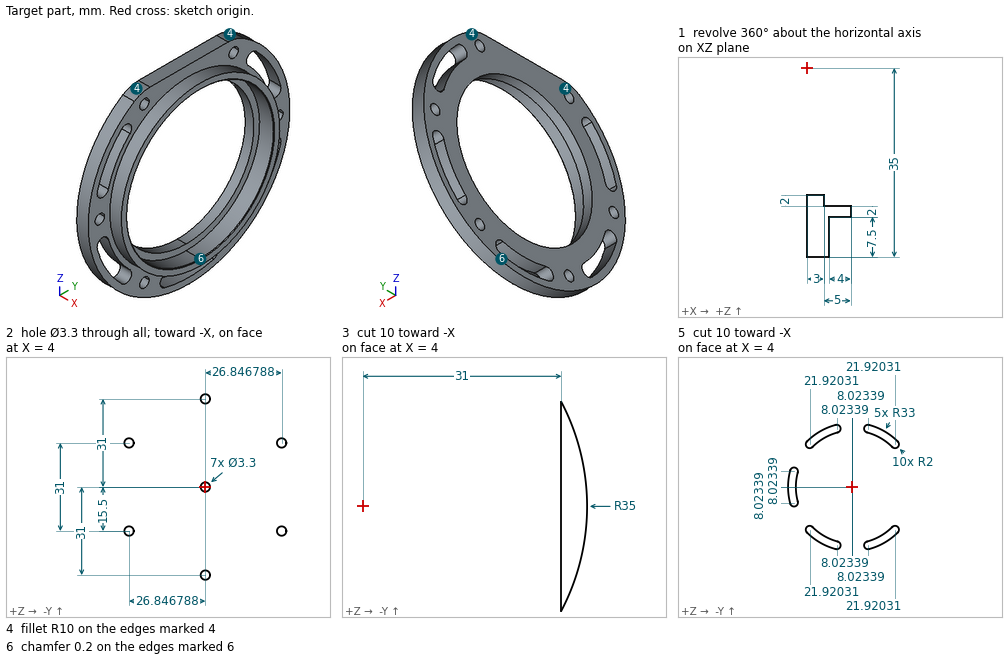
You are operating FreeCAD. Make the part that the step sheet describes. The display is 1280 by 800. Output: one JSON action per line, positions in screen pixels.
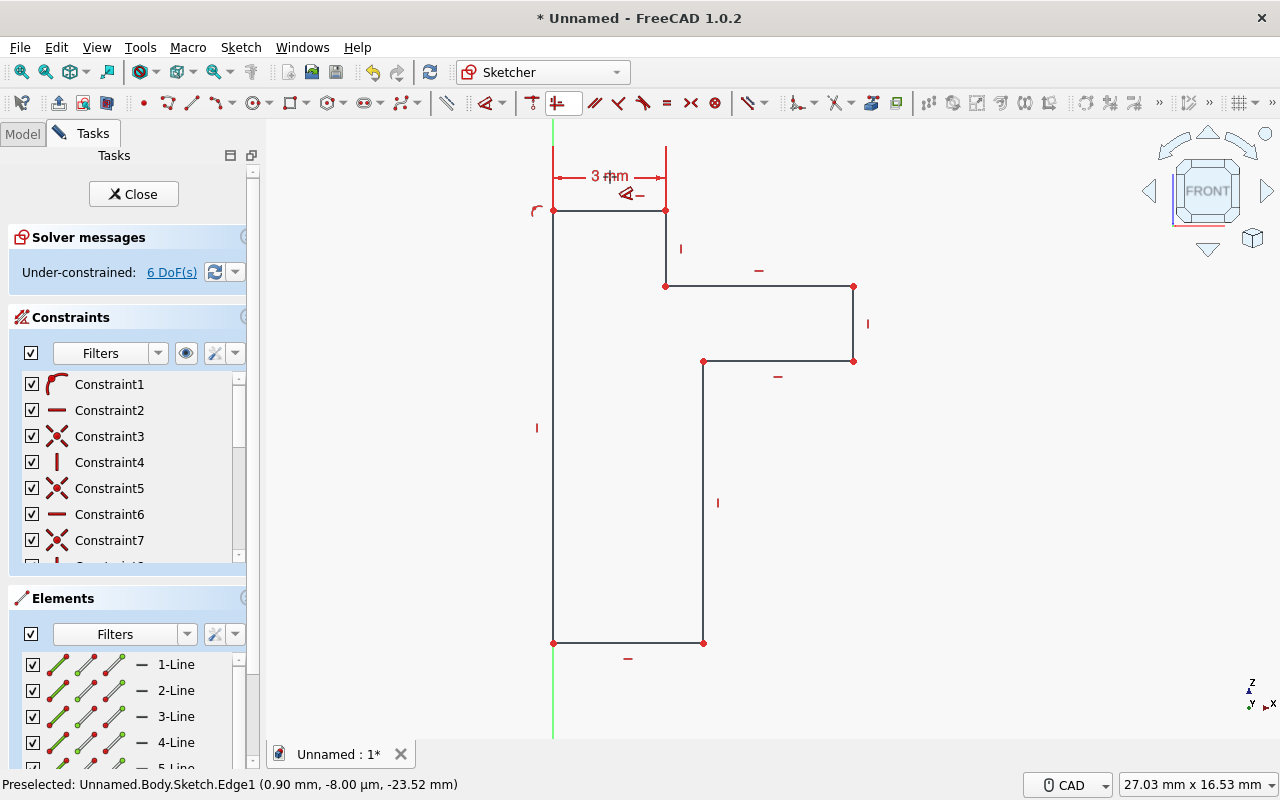
{"action": "left_click", "coordinate": [666, 233]}
{"action": "left_click", "coordinate": [632, 248]}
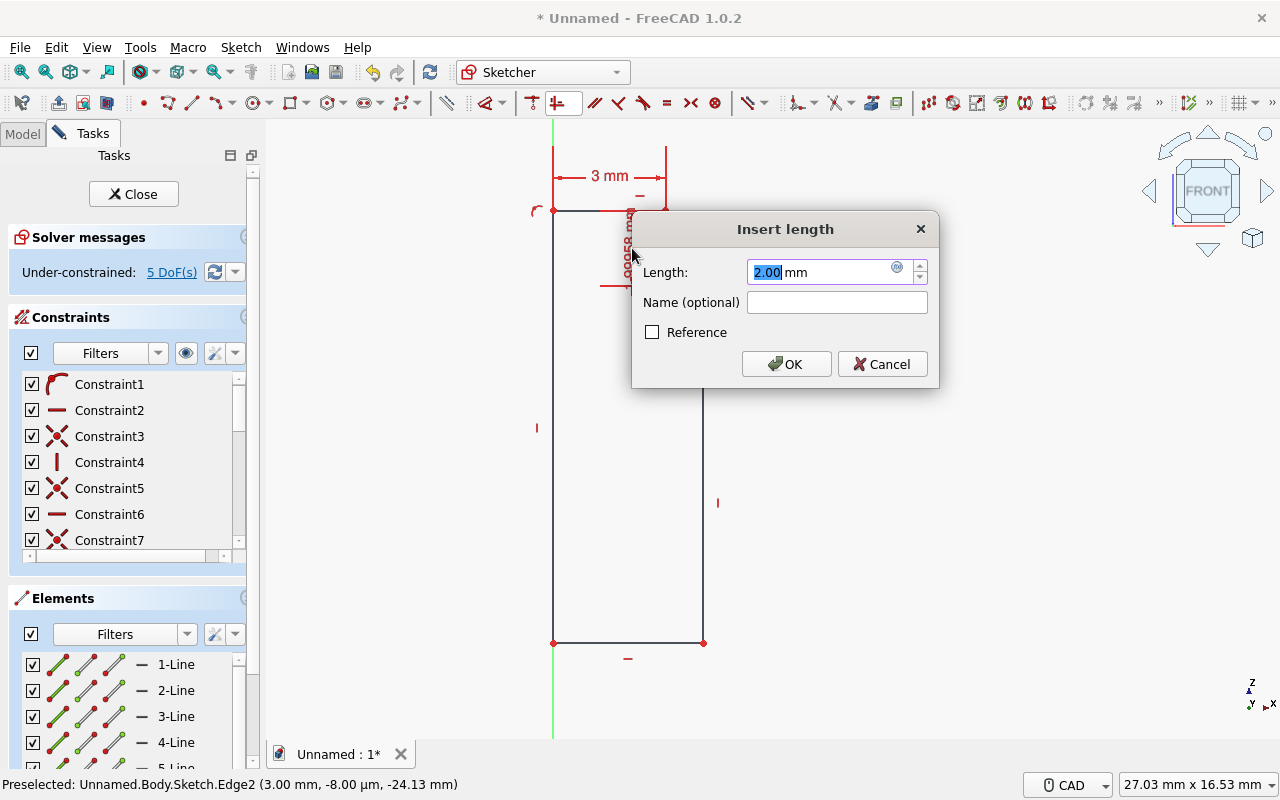
{"action": "type", "text": "2"}
{"action": "key", "text": "Return"}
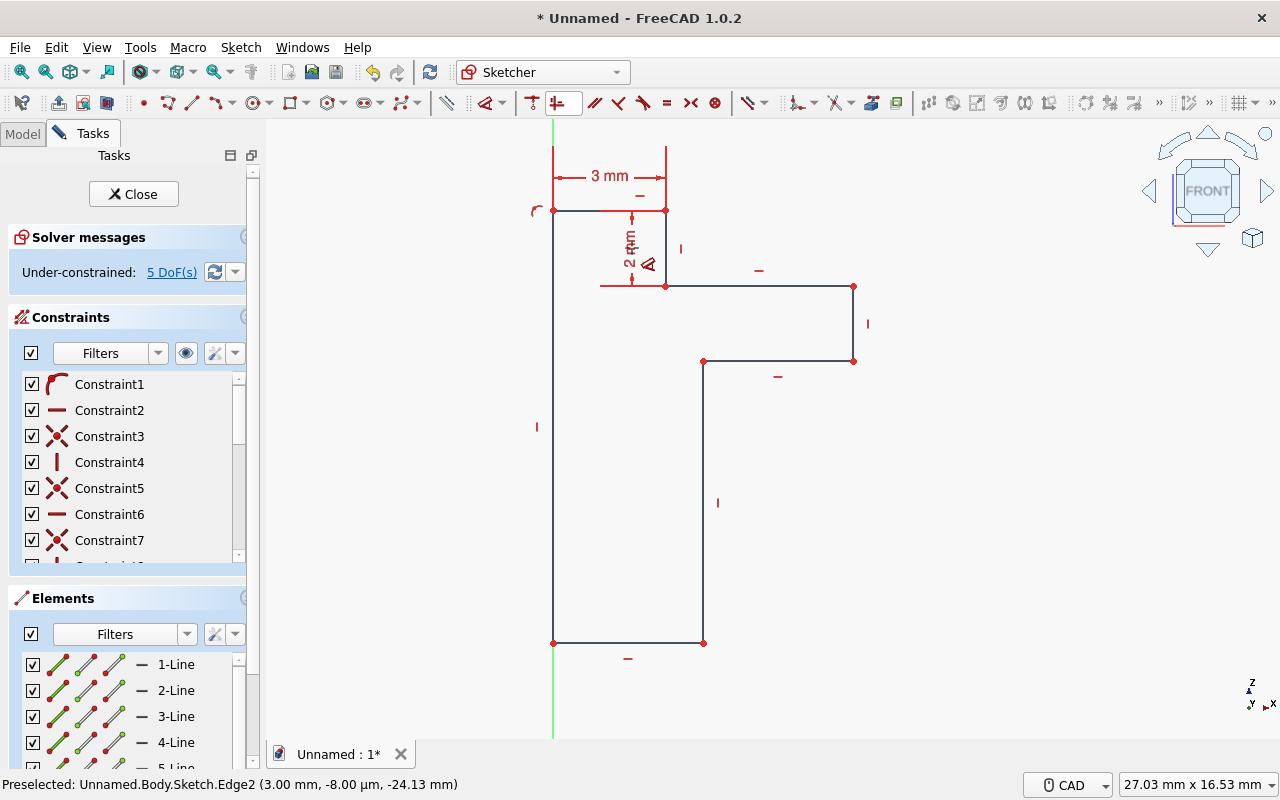
{"action": "left_click", "coordinate": [722, 286]}
{"action": "left_click", "coordinate": [759, 252]}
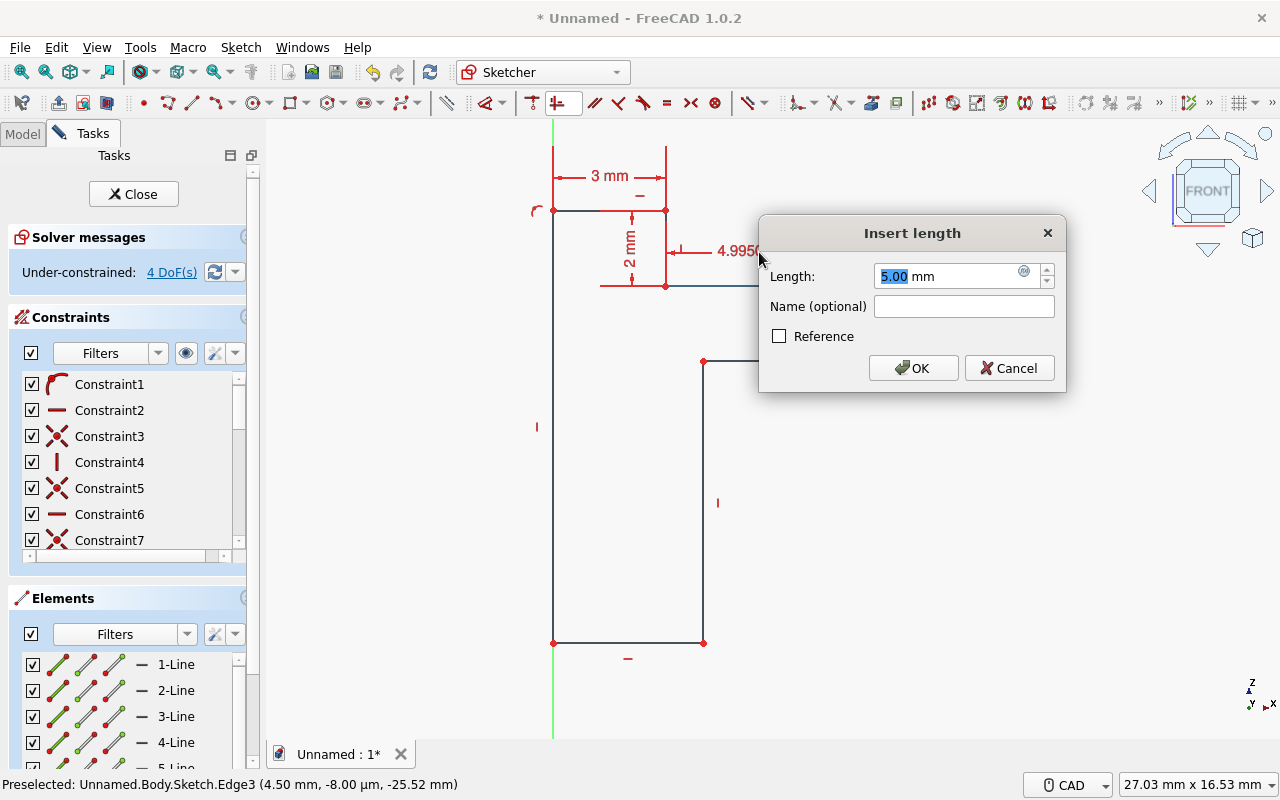
{"action": "type", "text": "5"}
{"action": "key", "text": "Return"}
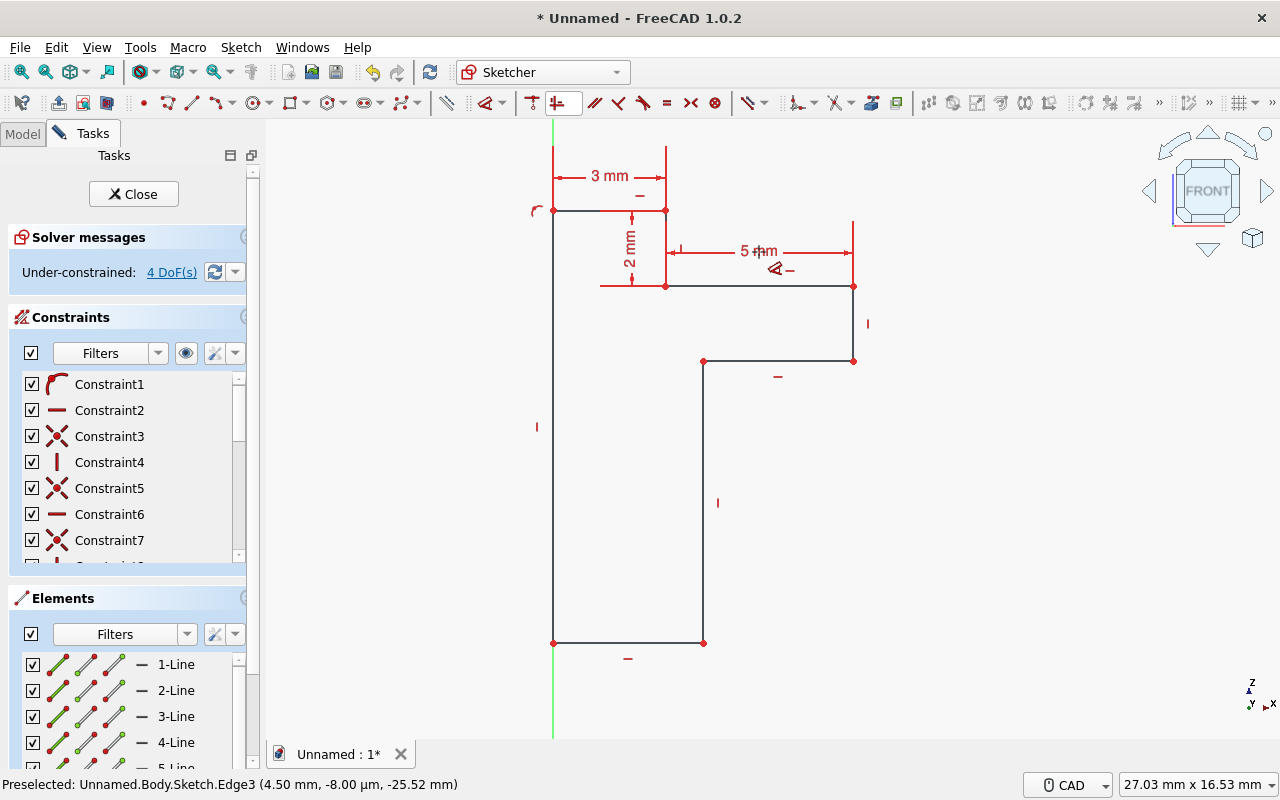
{"action": "left_click", "coordinate": [853, 308]}
{"action": "left_click", "coordinate": [887, 323]}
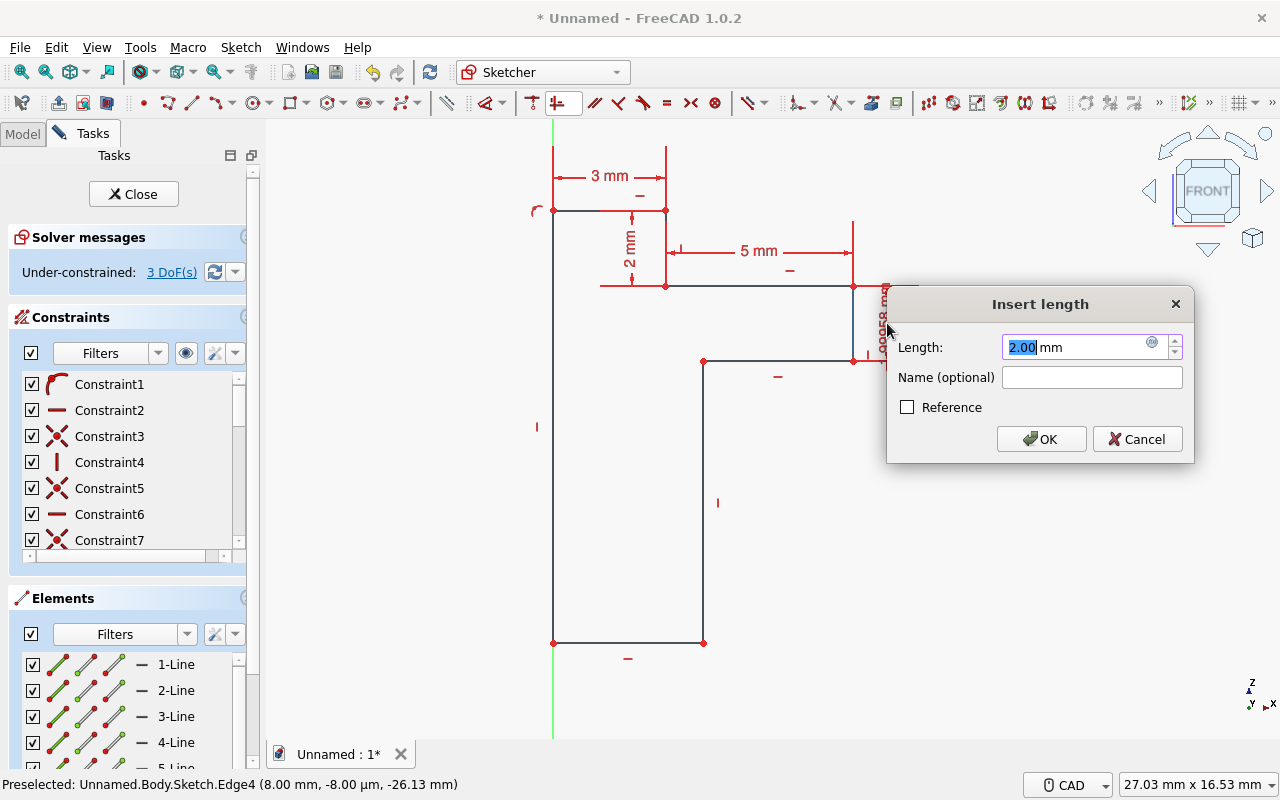
{"action": "type", "text": "2"}
{"action": "key", "text": "Return"}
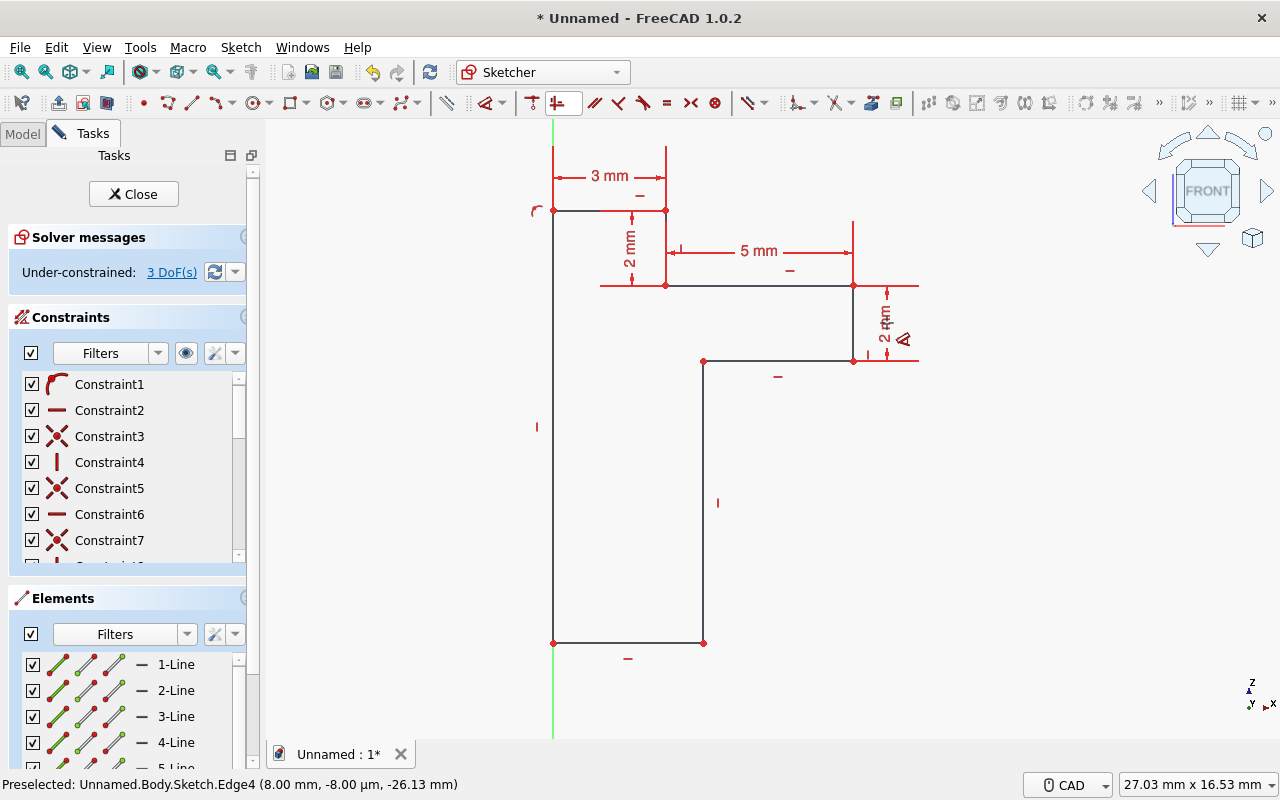
{"action": "left_click", "coordinate": [808, 361]}
{"action": "left_click", "coordinate": [778, 327]}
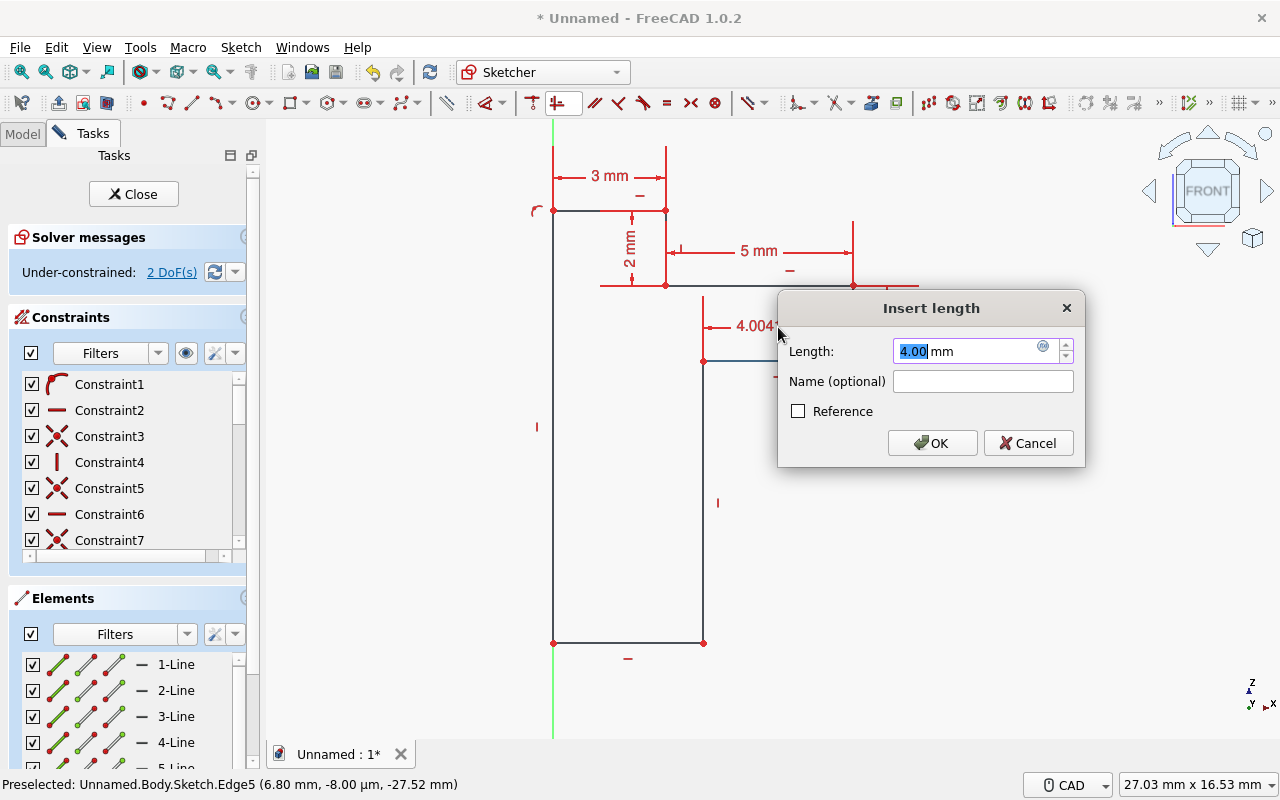
{"action": "type", "text": "4"}
{"action": "key", "text": "Return"}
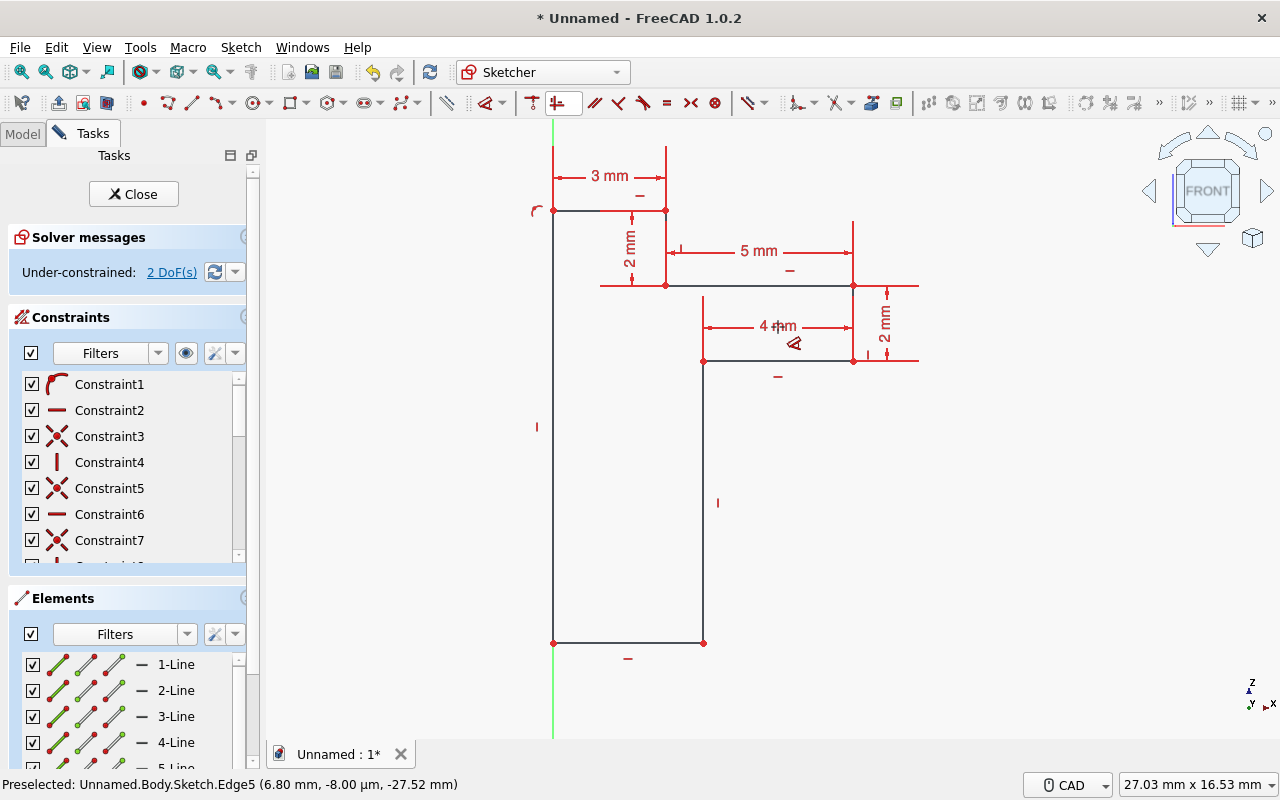
{"action": "left_click", "coordinate": [703, 446]}
{"action": "left_click", "coordinate": [737, 502]}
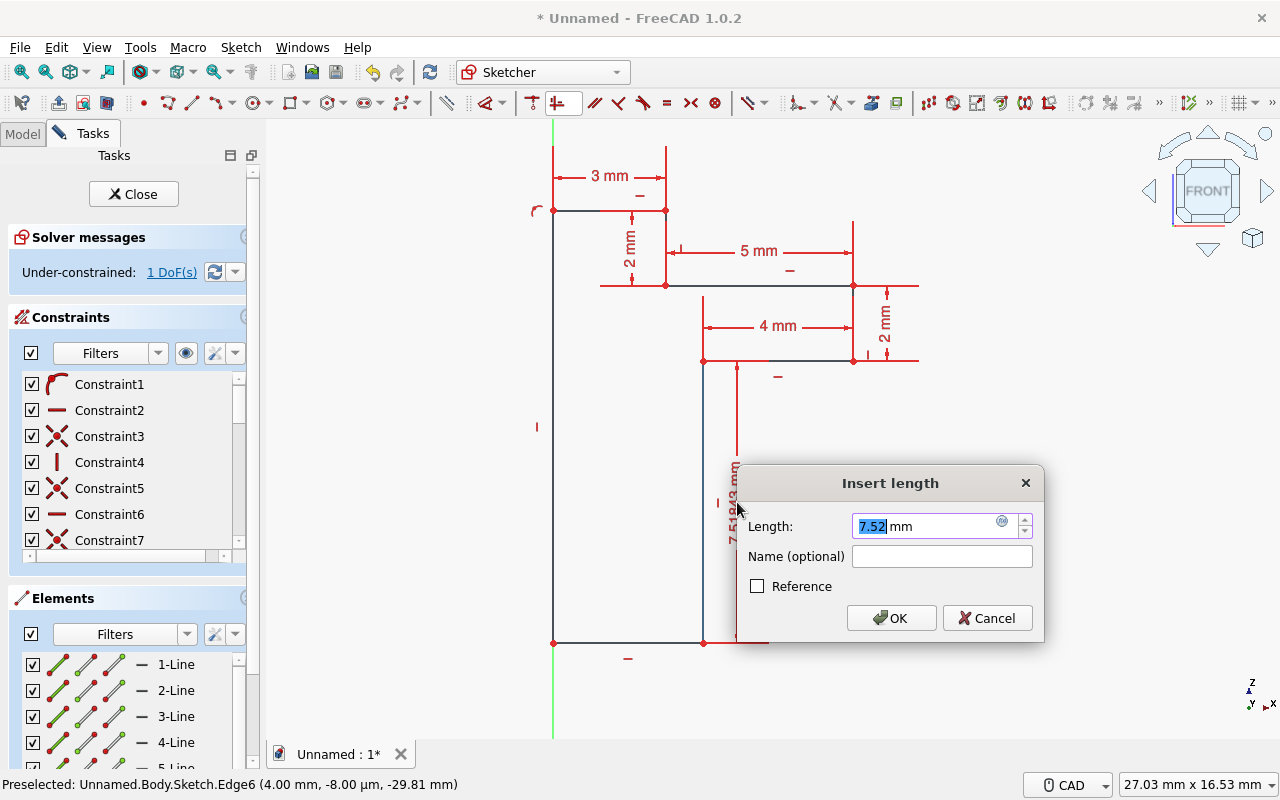
{"action": "type", "text": "7.5"}
{"action": "key", "text": "Return"}